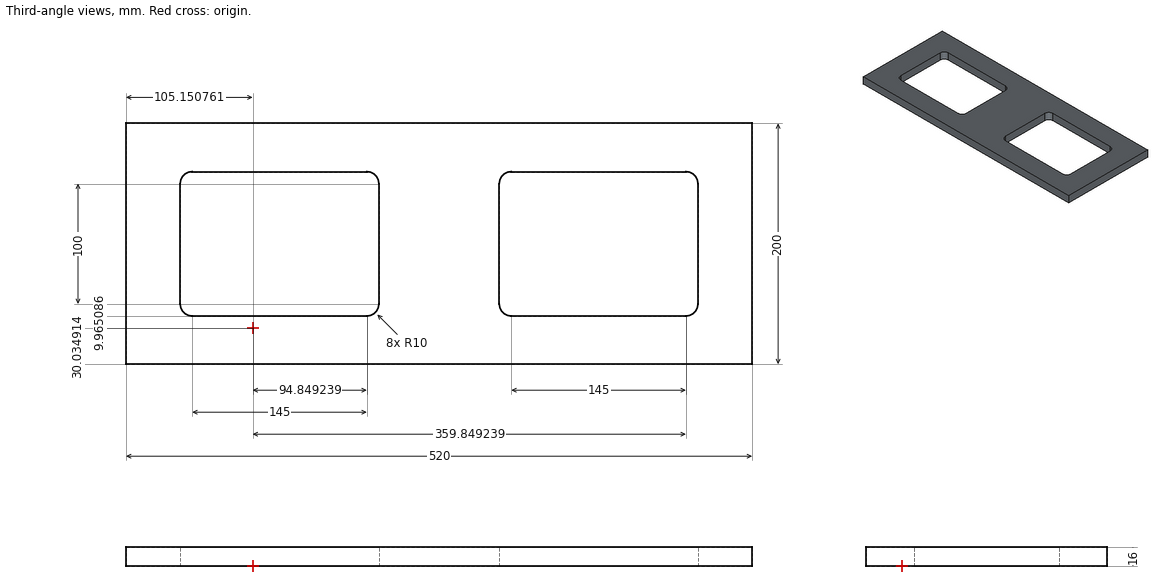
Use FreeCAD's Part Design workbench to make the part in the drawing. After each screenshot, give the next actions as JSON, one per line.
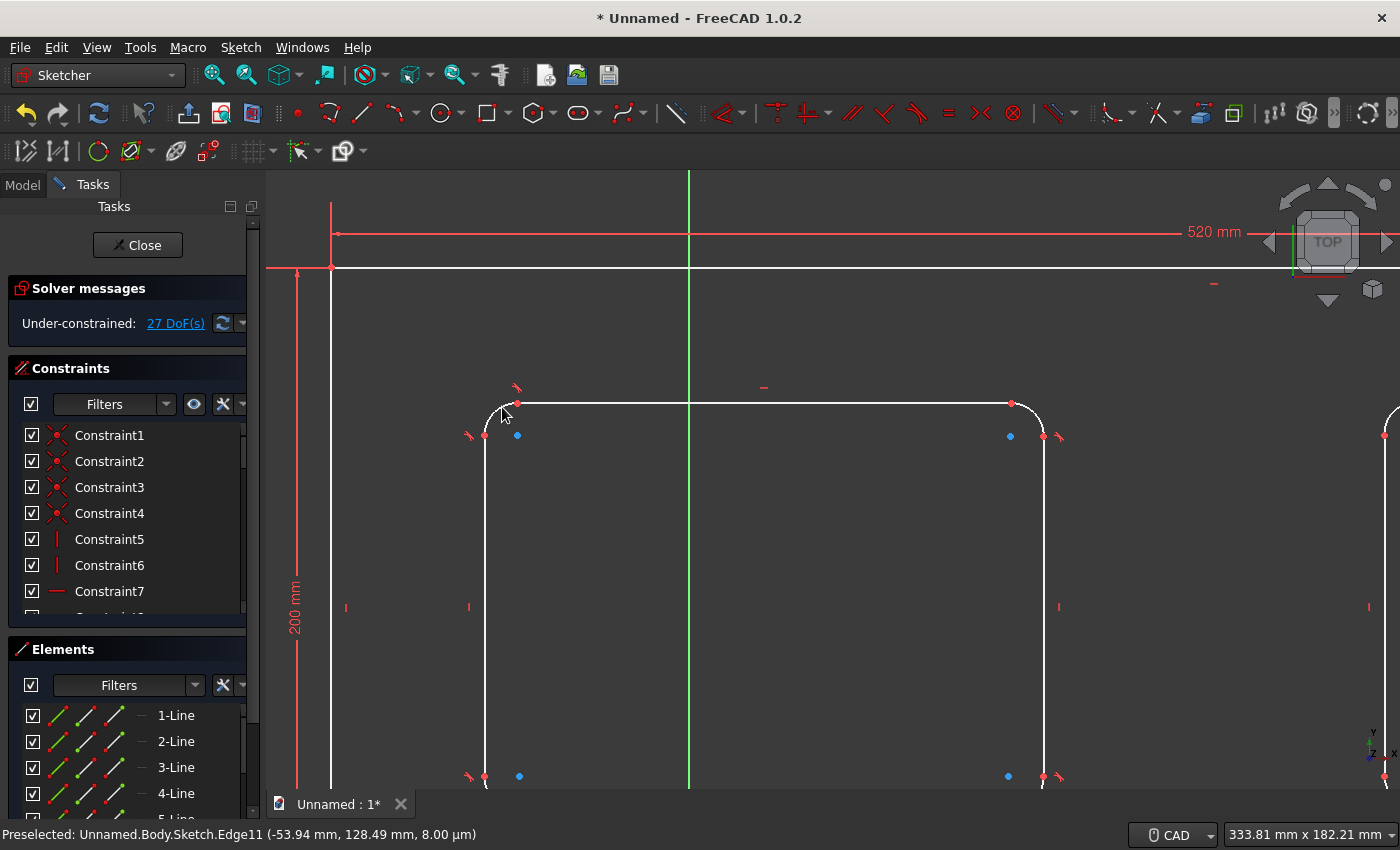
{"action": "left_click", "coordinate": [666, 403]}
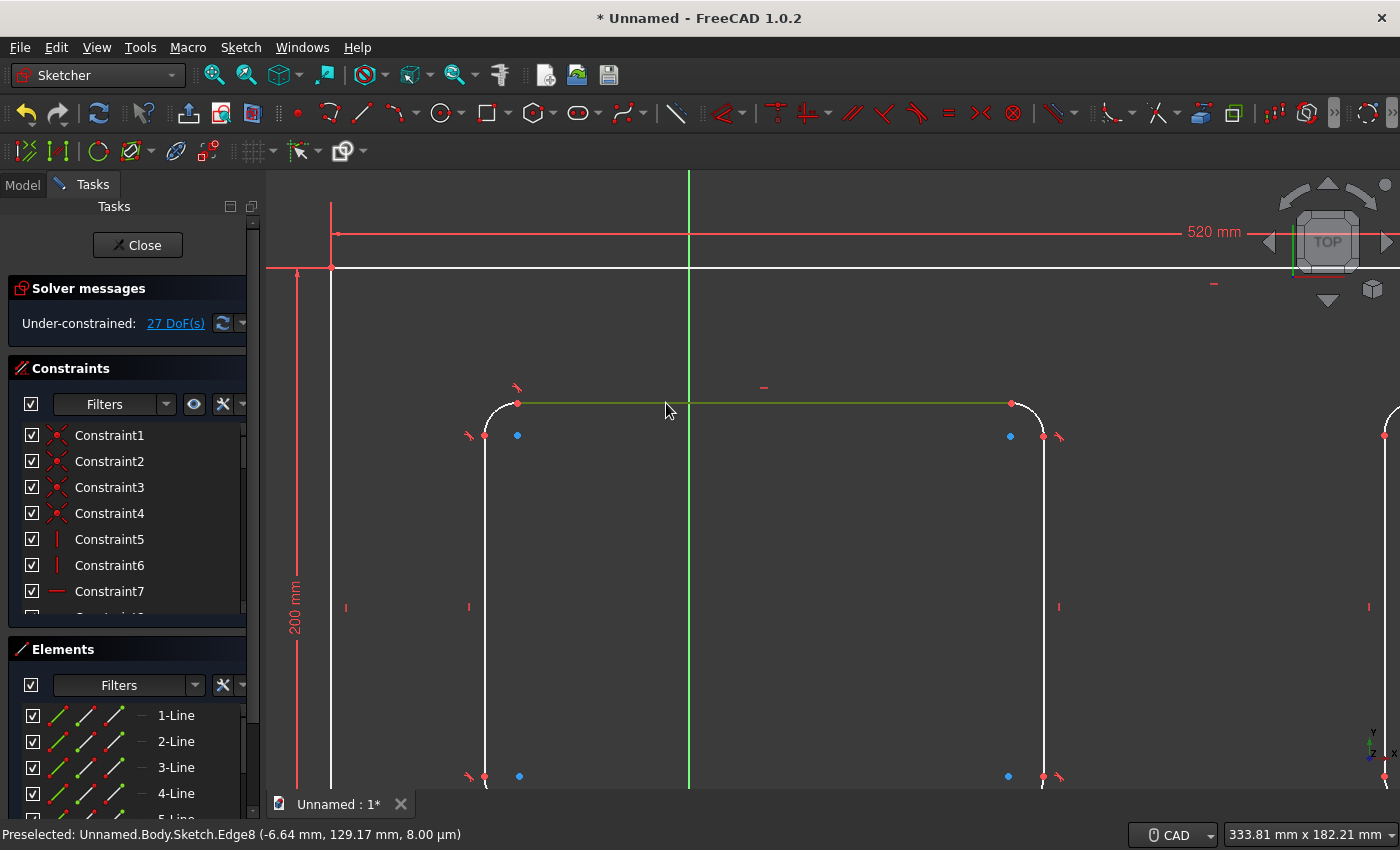
{"action": "left_click", "coordinate": [1040, 421]}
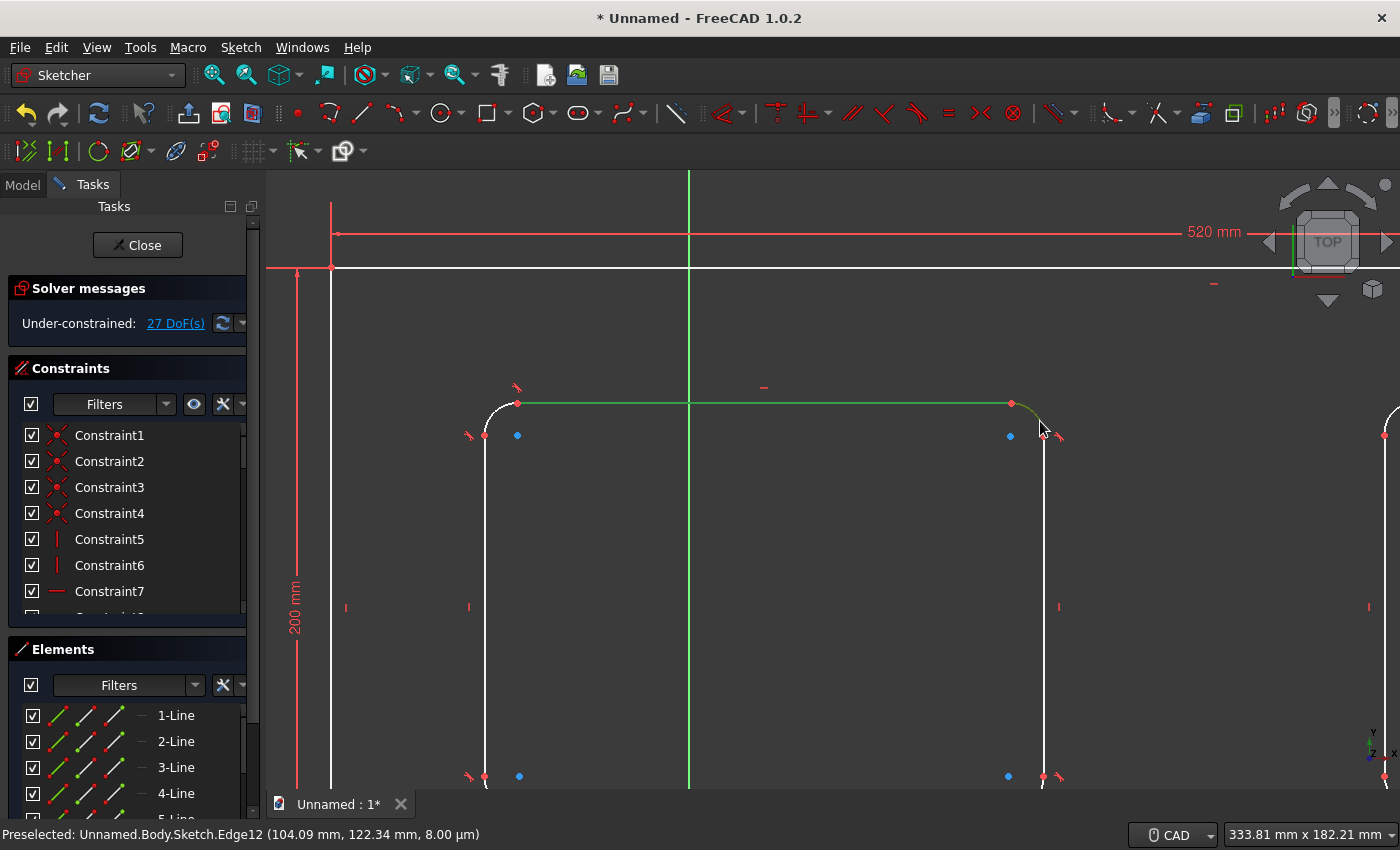
{"action": "left_click", "coordinate": [918, 114]}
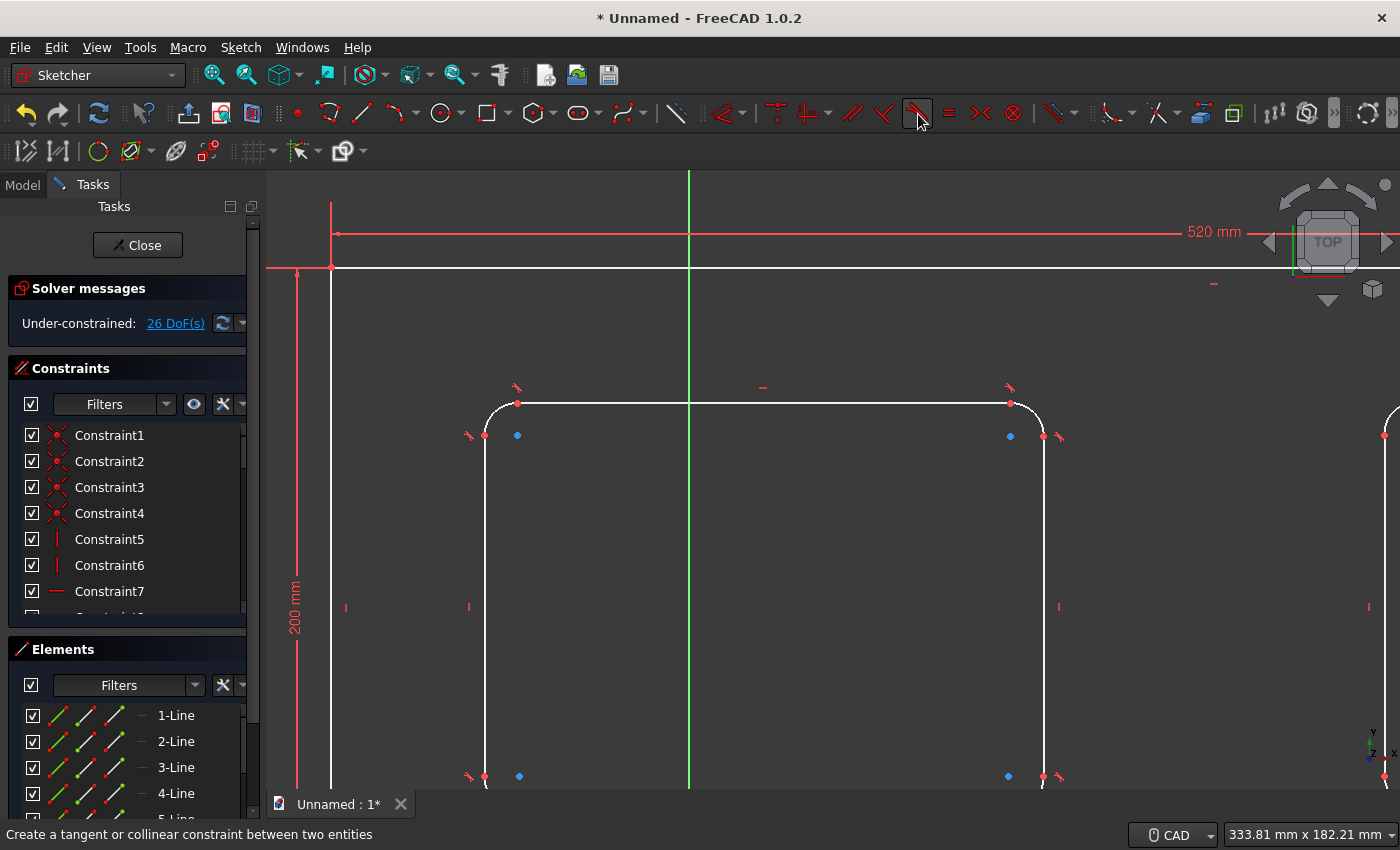
{"action": "scroll", "coordinate": [503, 407], "scroll_direction": "down", "scroll_amount": 5}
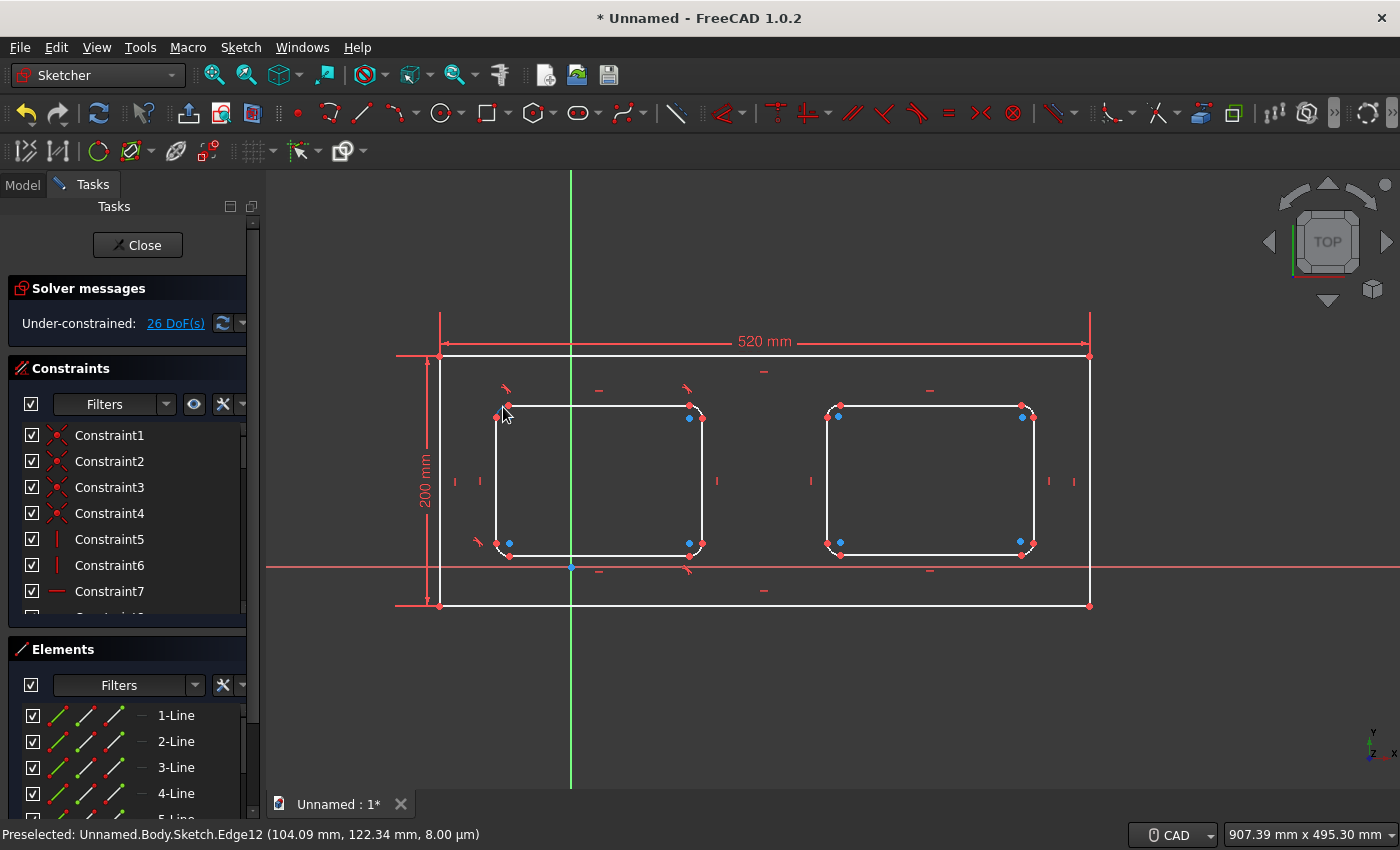
{"action": "left_click", "coordinate": [967, 555]}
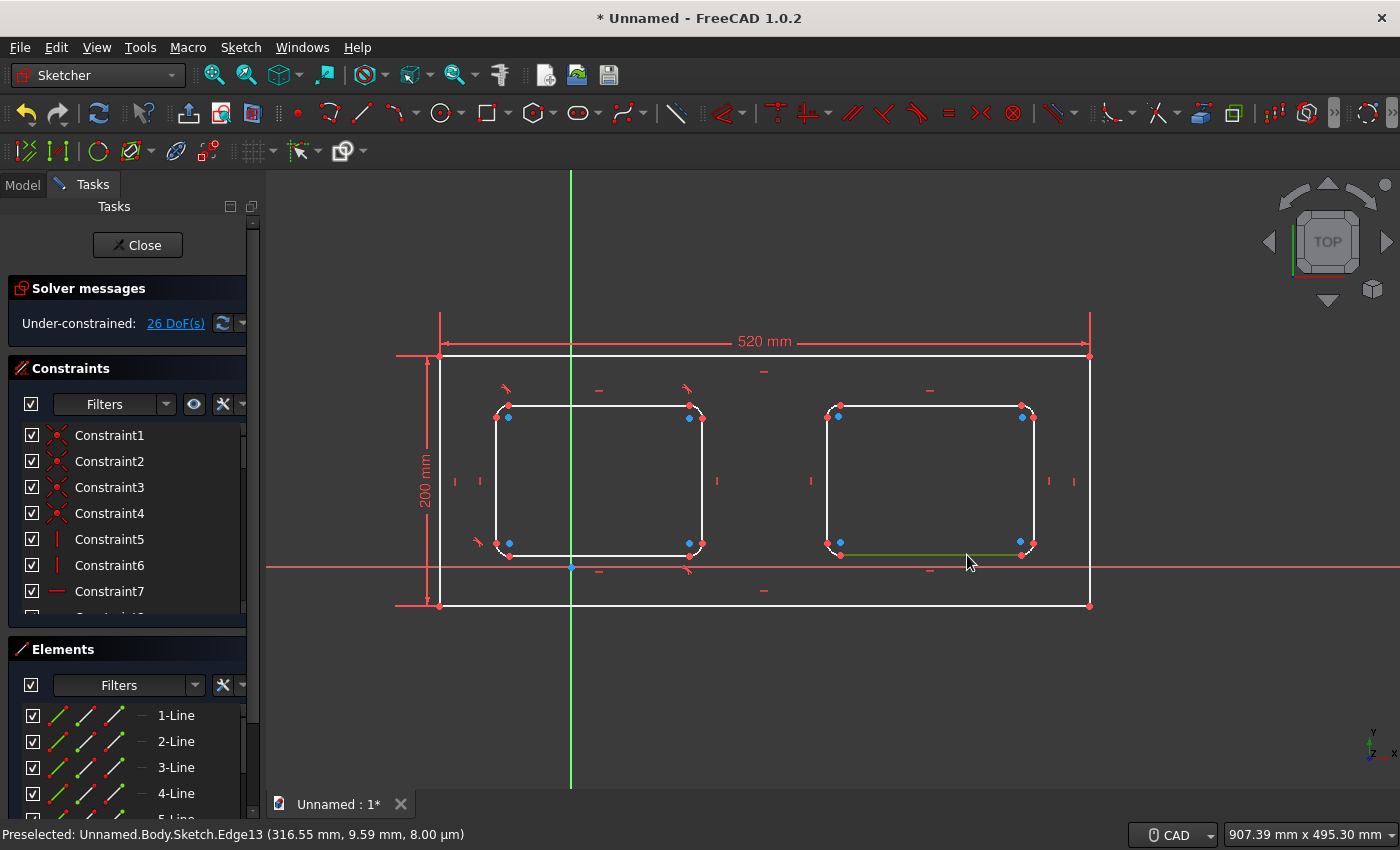
{"action": "scroll", "coordinate": [831, 552], "scroll_direction": "up", "scroll_amount": 2}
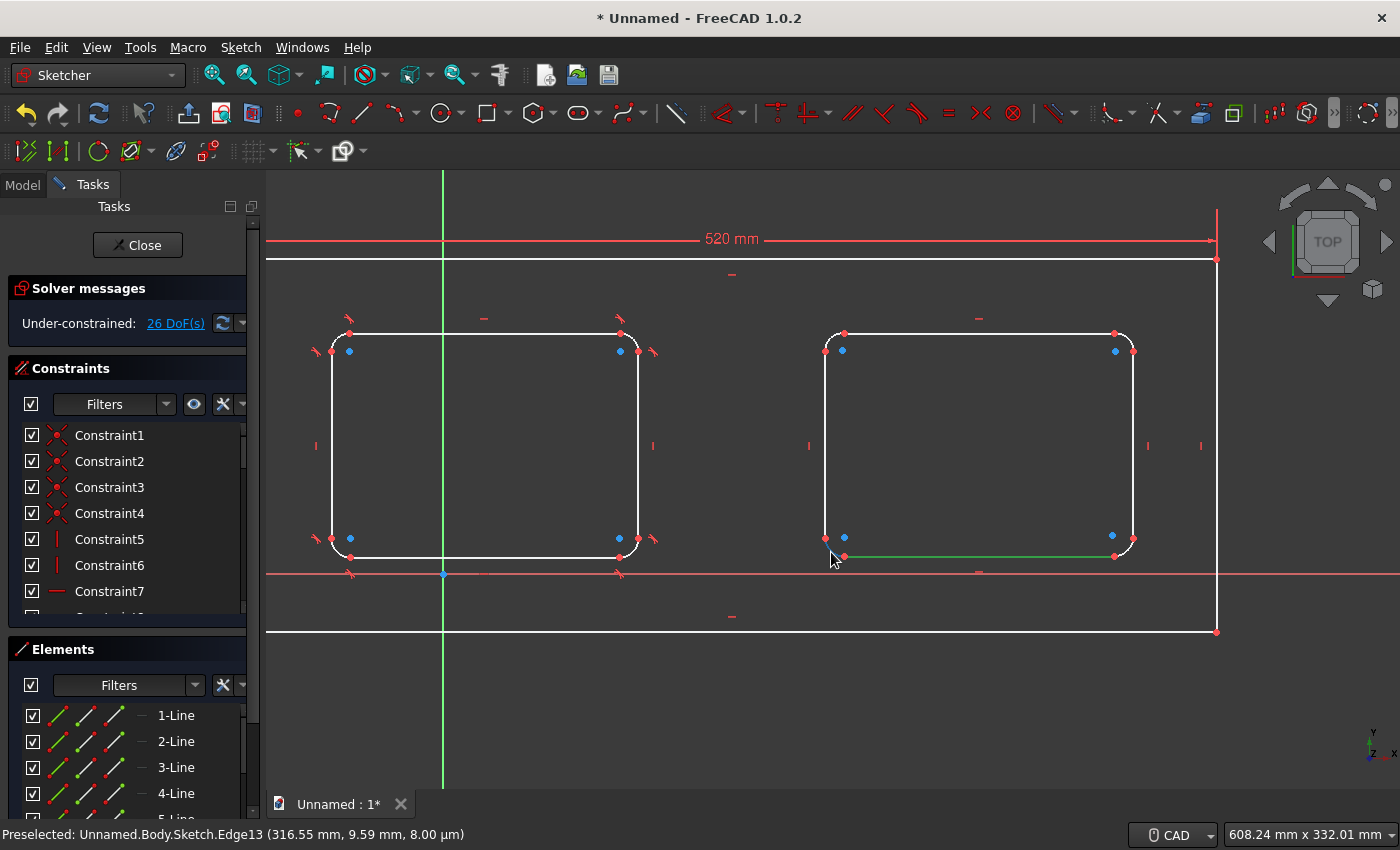
{"action": "left_click", "coordinate": [831, 551]}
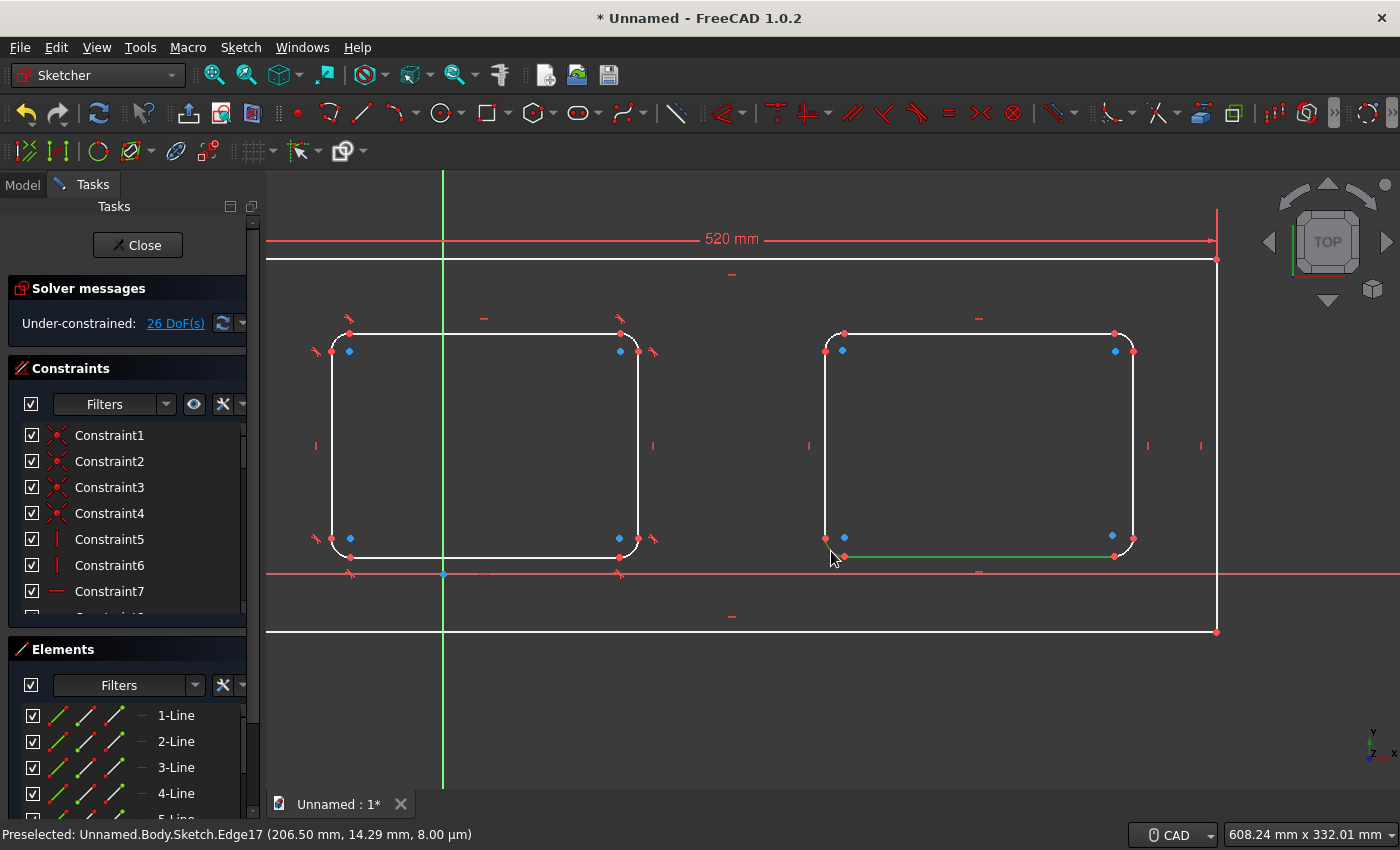
{"action": "left_click", "coordinate": [918, 114]}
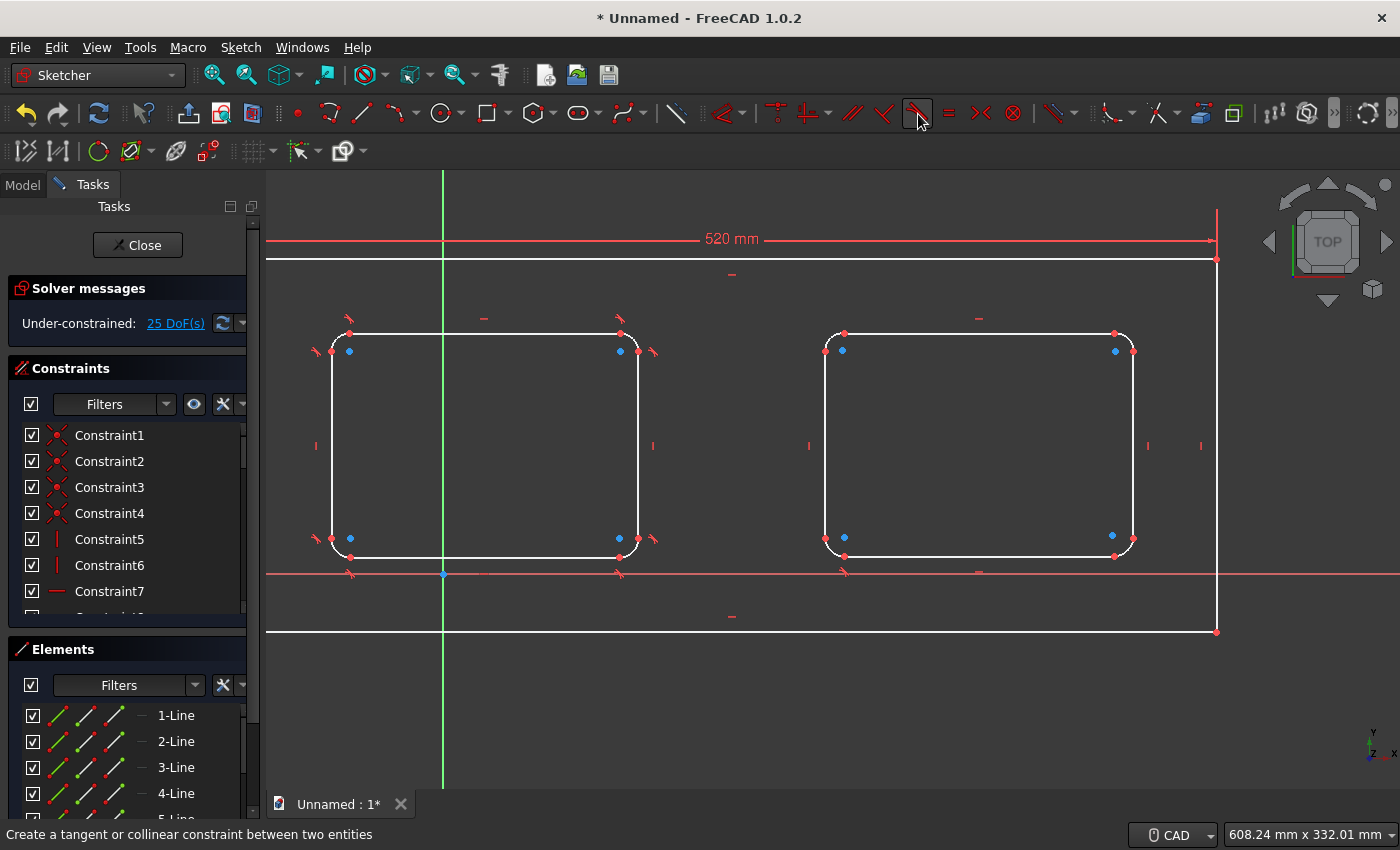
{"action": "left_click", "coordinate": [1033, 557]}